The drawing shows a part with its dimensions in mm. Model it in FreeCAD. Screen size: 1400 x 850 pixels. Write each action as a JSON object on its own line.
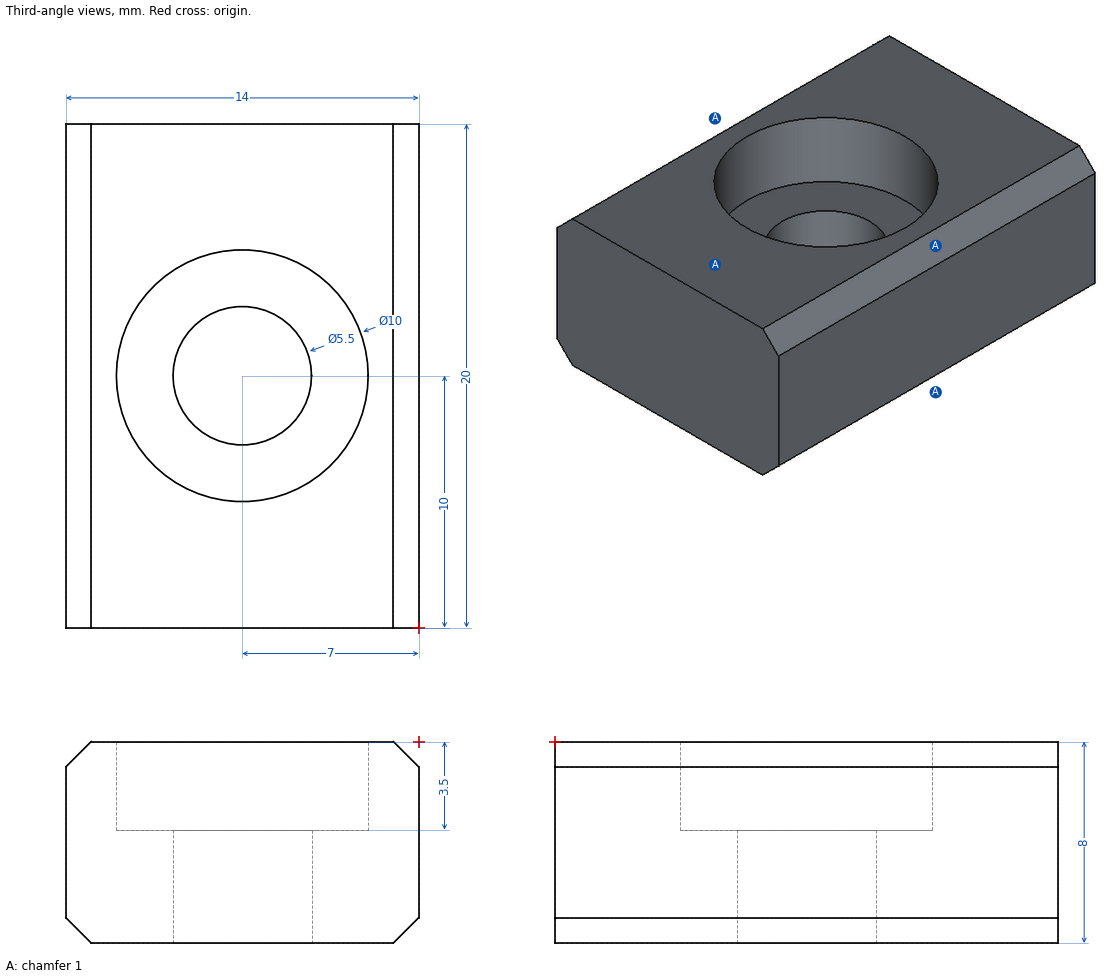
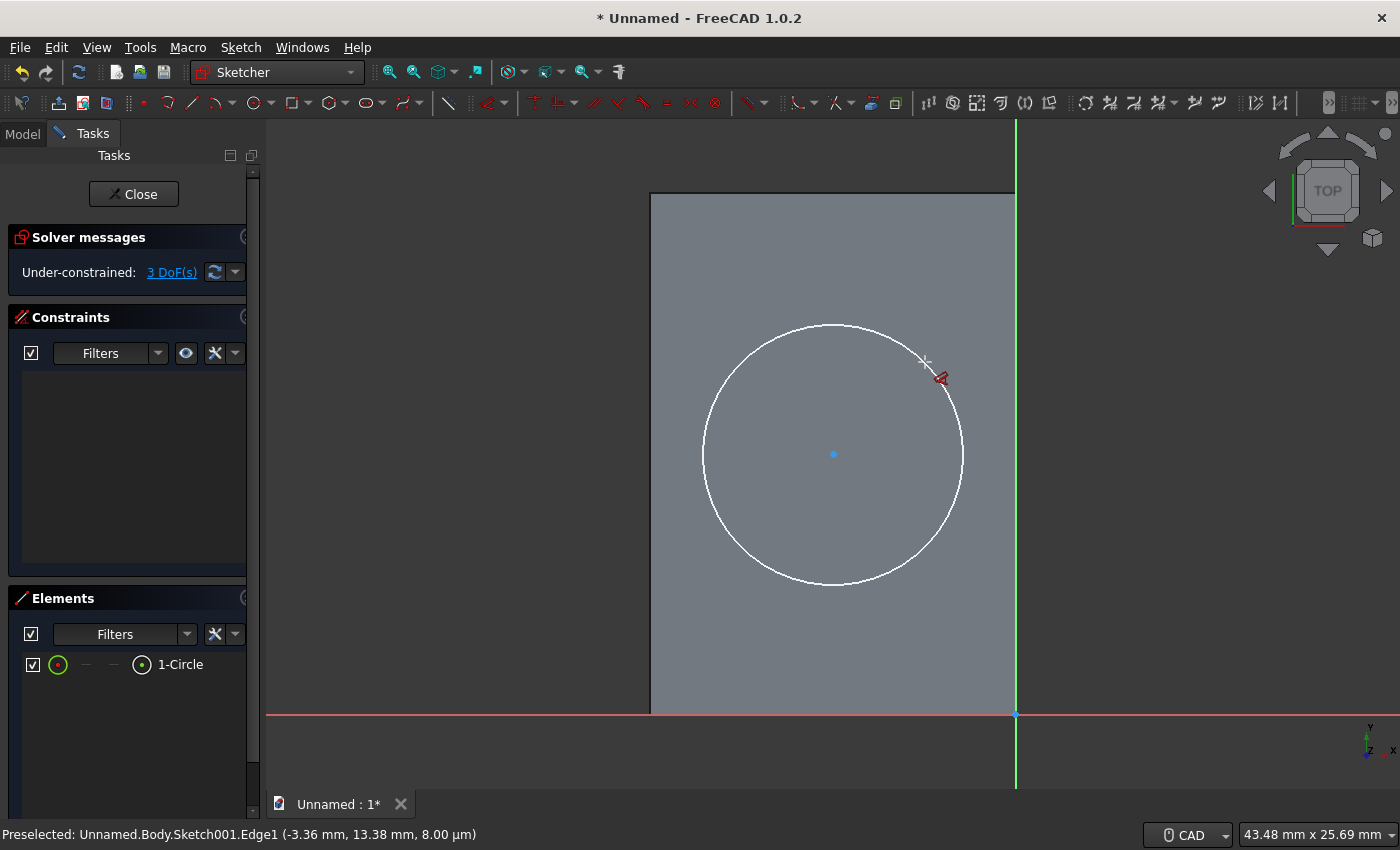
{"action": "left_click", "coordinate": [925, 363]}
{"action": "left_click", "coordinate": [948, 340]}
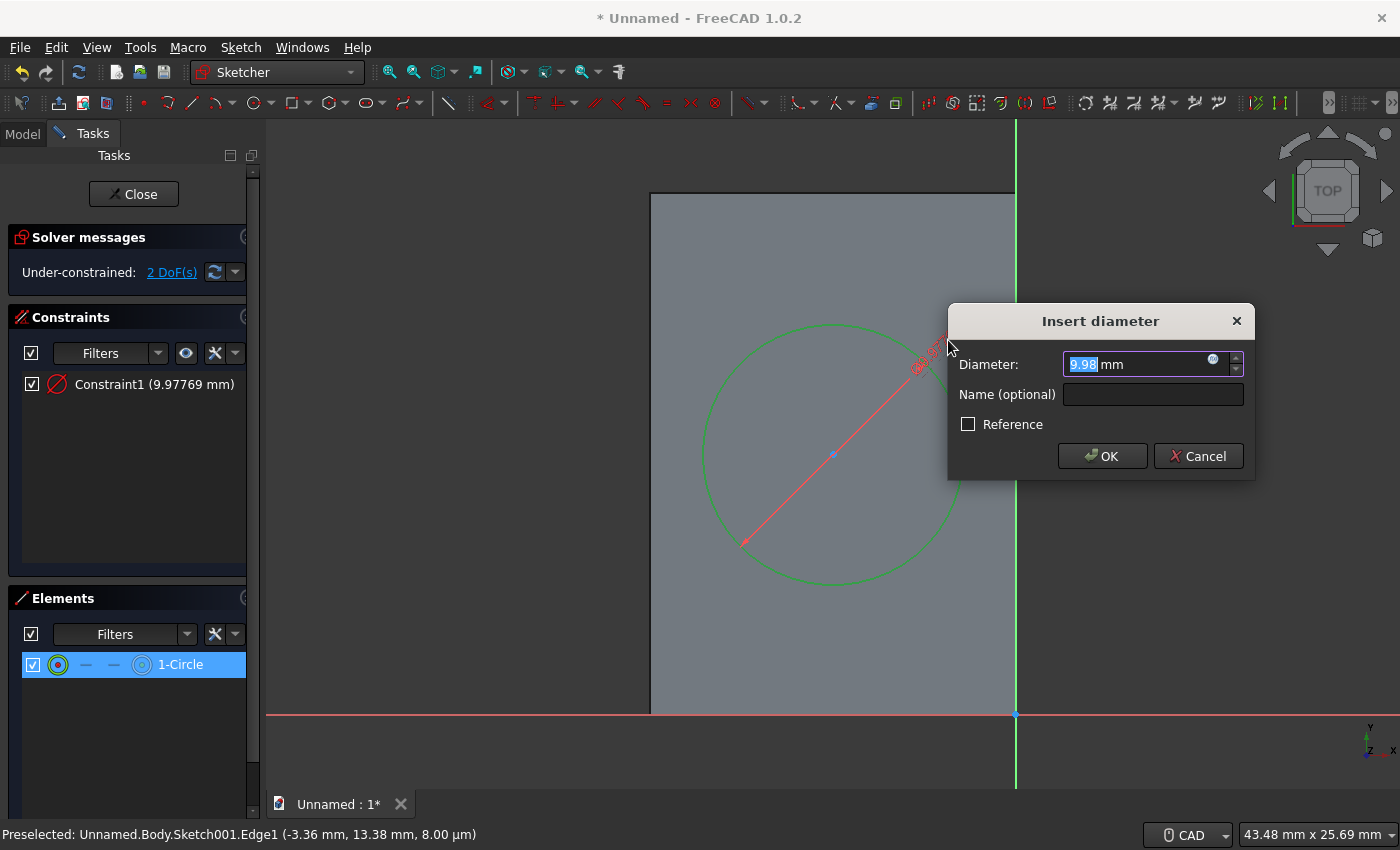
{"action": "type", "text": "10"}
{"action": "key", "text": "Return"}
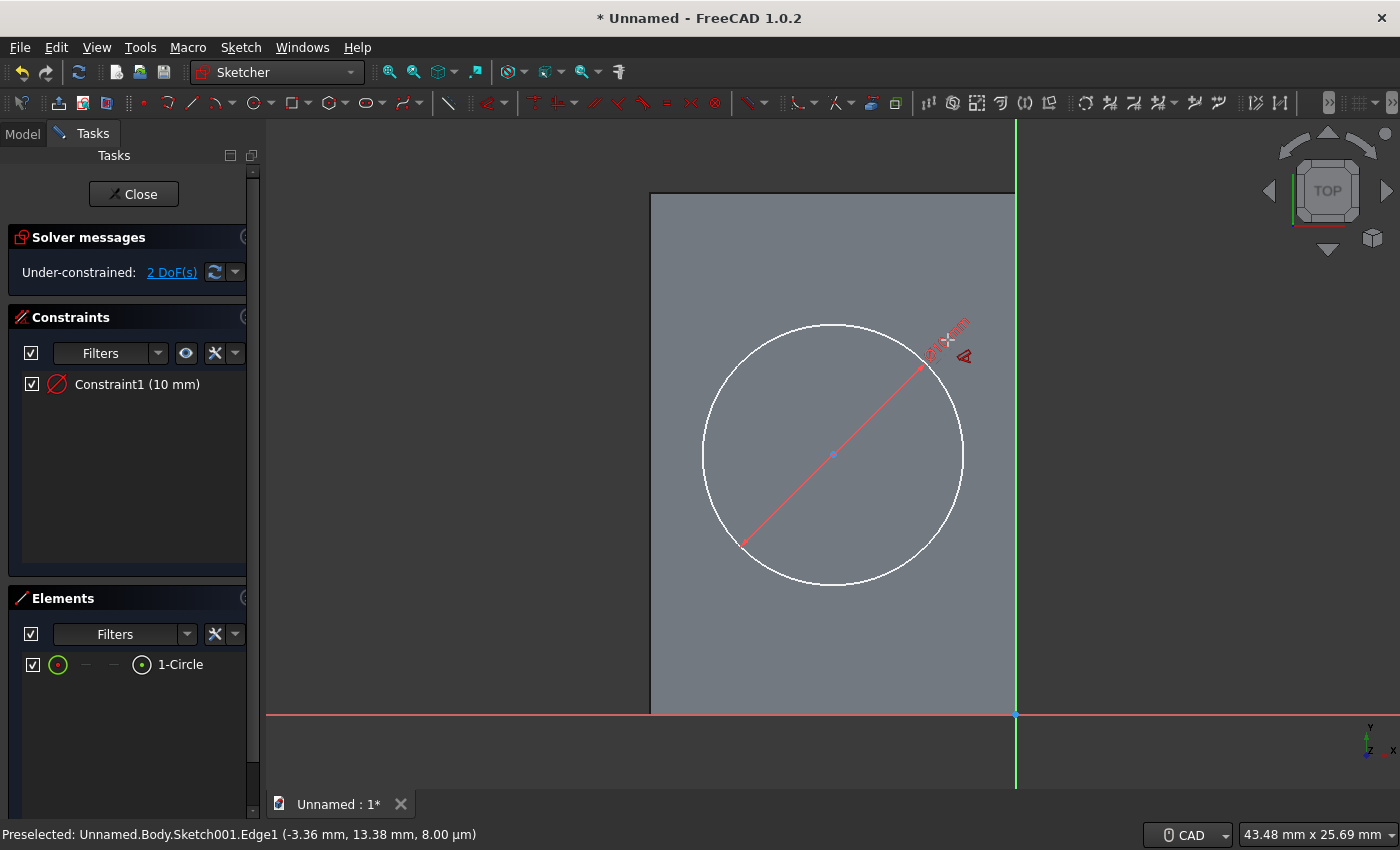
{"action": "left_click", "coordinate": [833, 455]}
{"action": "left_click", "coordinate": [924, 749]}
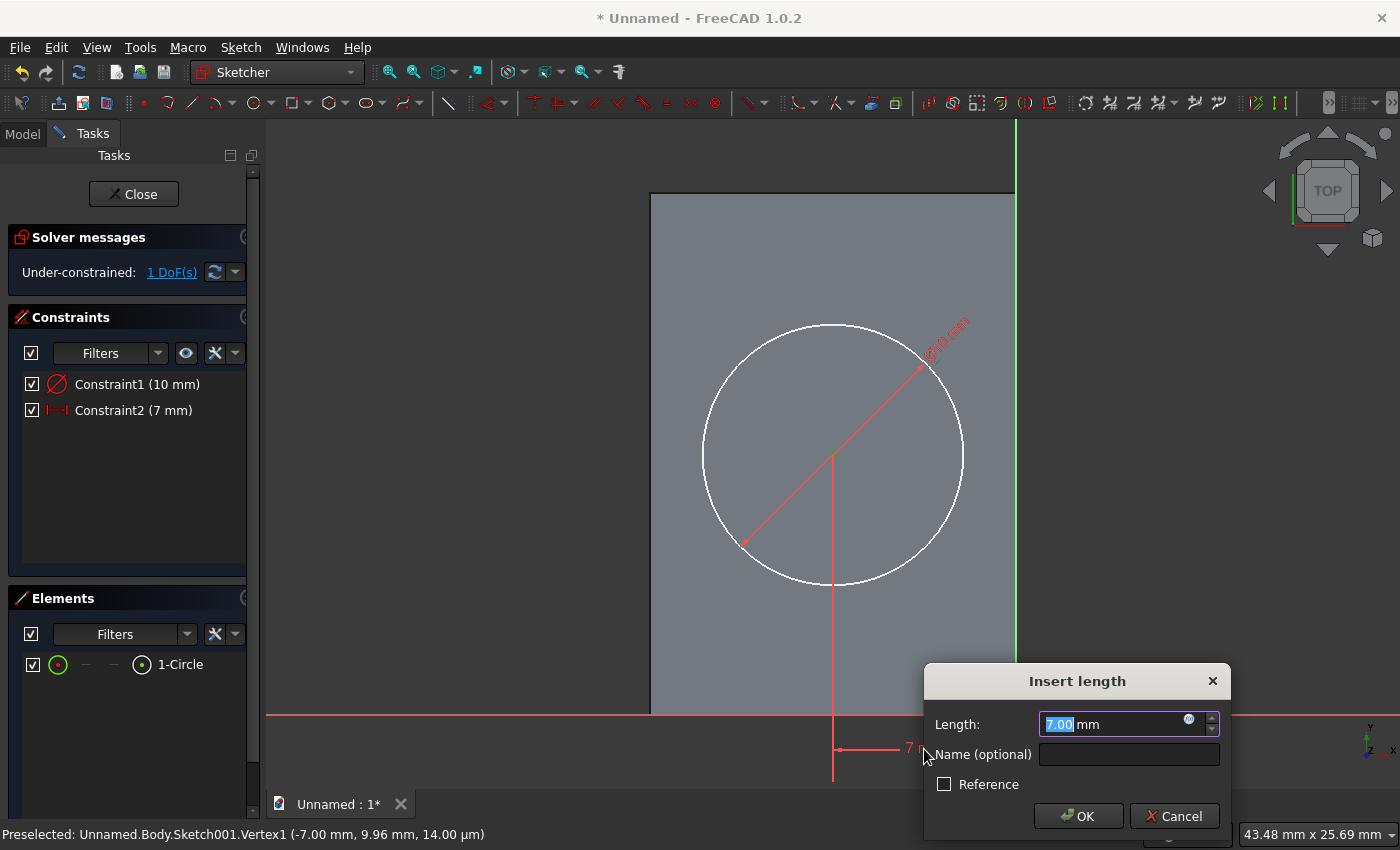
{"action": "type", "text": "7"}
{"action": "key", "text": "Return"}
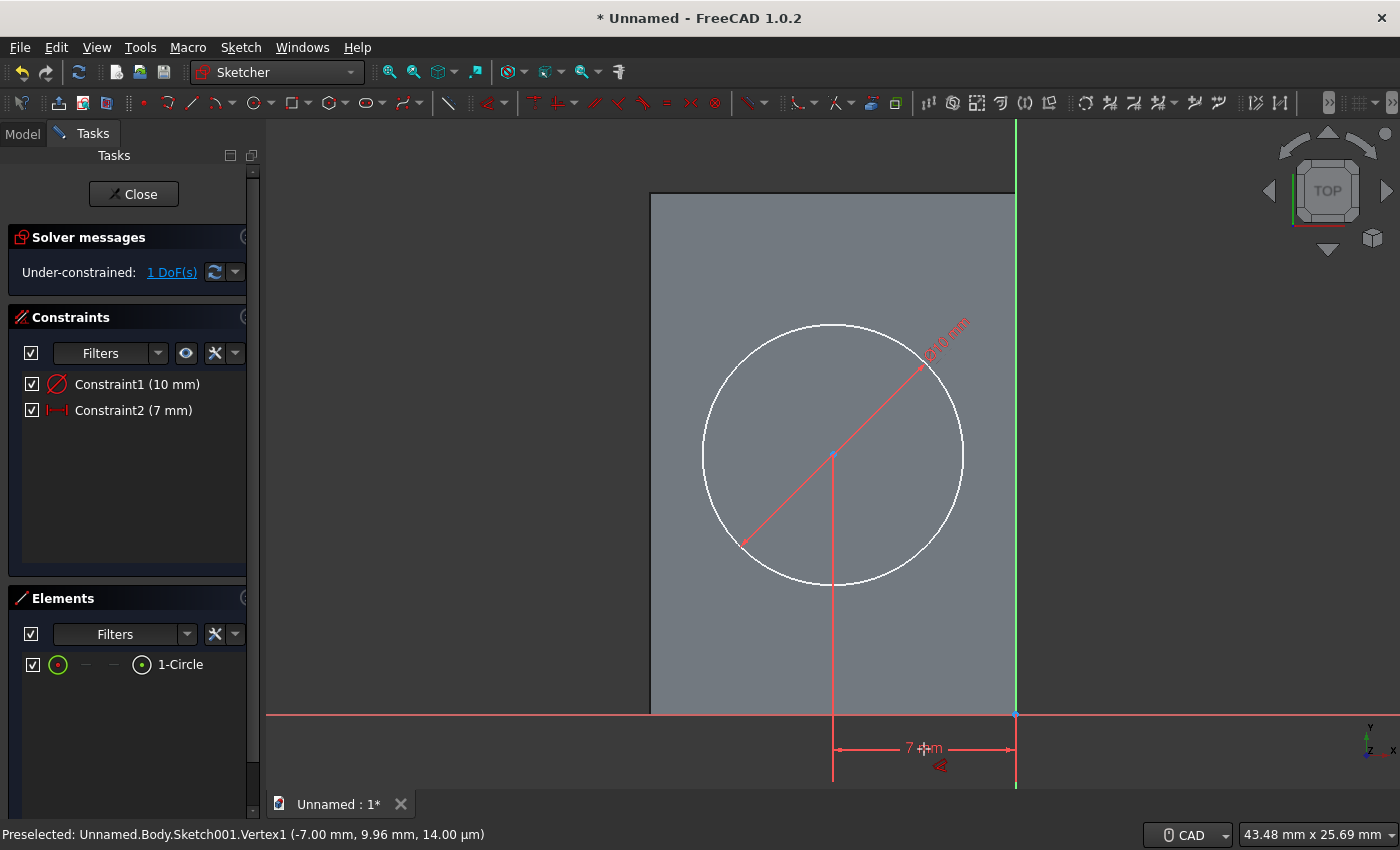
{"action": "left_click", "coordinate": [833, 455]}
{"action": "left_click", "coordinate": [1050, 585]}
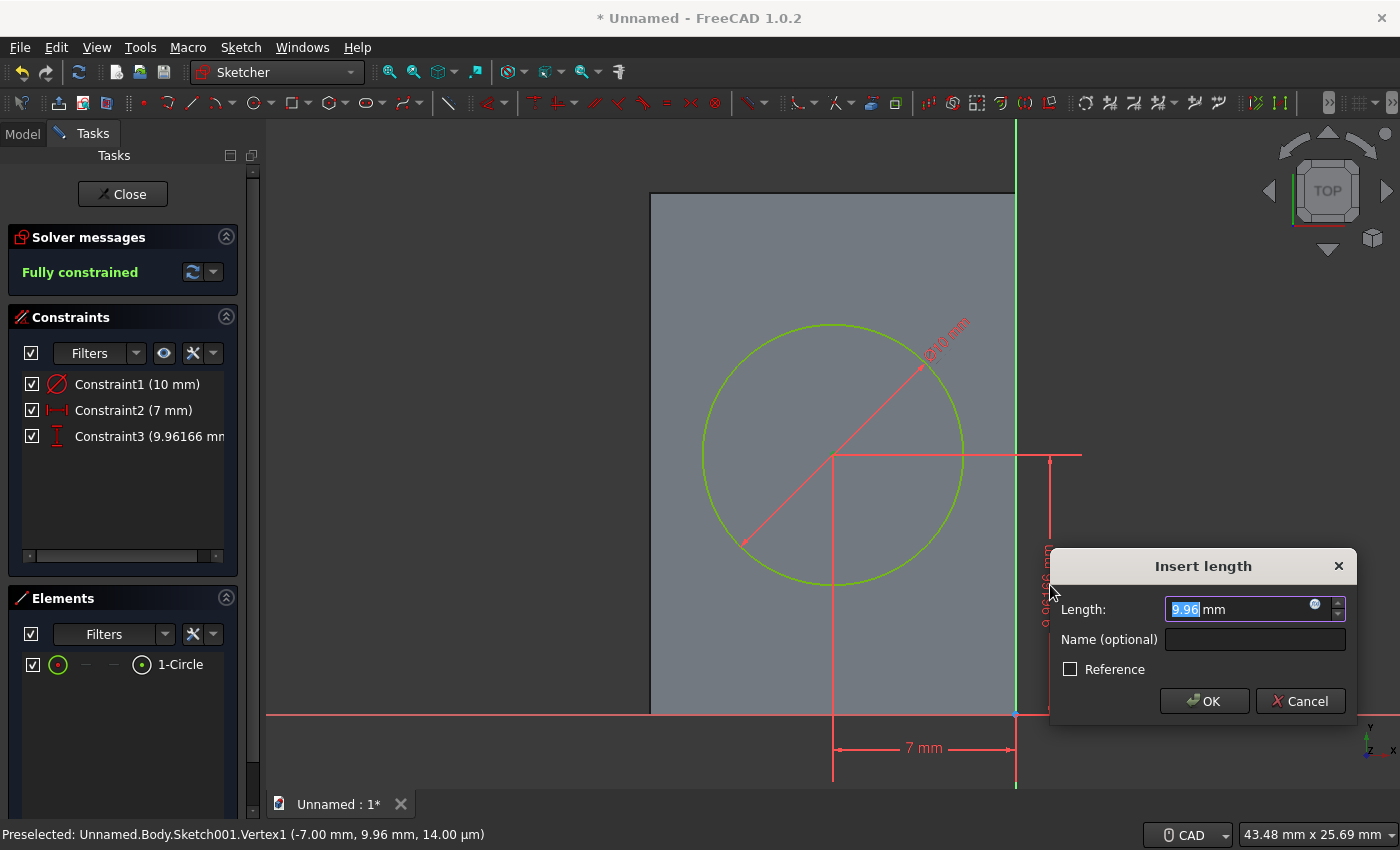
{"action": "type", "text": "10"}
{"action": "key", "text": "Return"}
{"action": "key", "text": "Escape"}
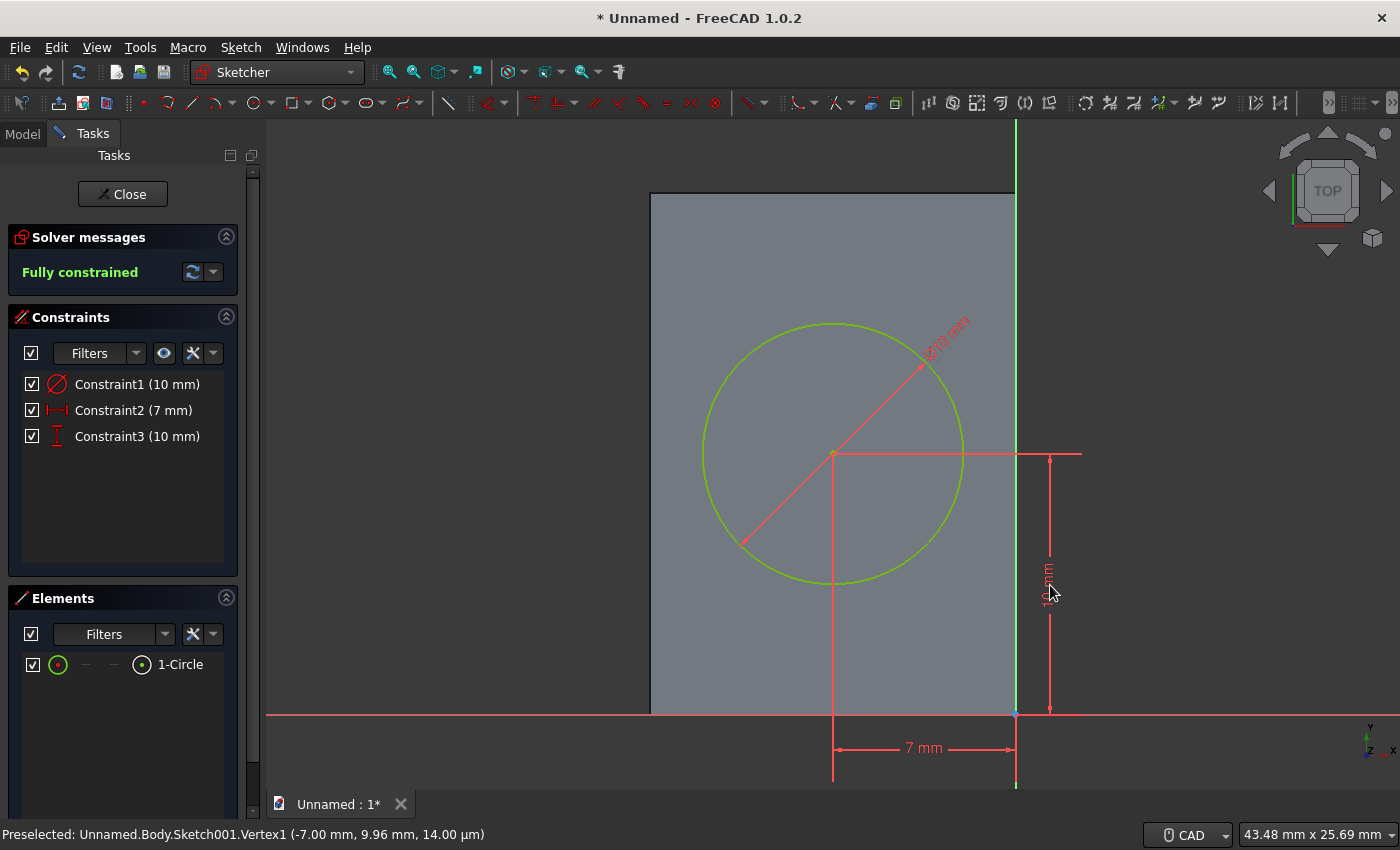
{"action": "left_click", "coordinate": [123, 194]}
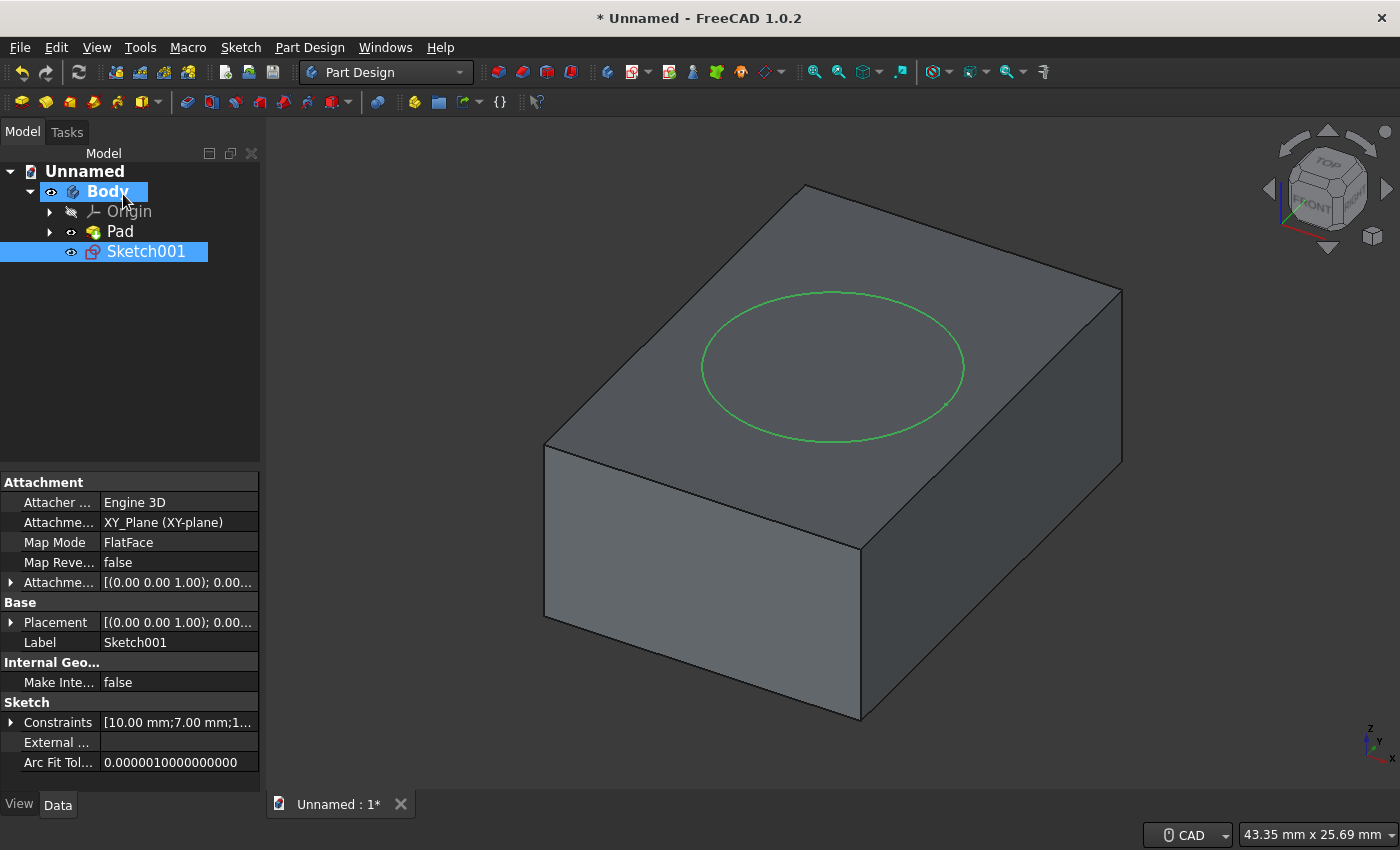
{"action": "left_click", "coordinate": [188, 102]}